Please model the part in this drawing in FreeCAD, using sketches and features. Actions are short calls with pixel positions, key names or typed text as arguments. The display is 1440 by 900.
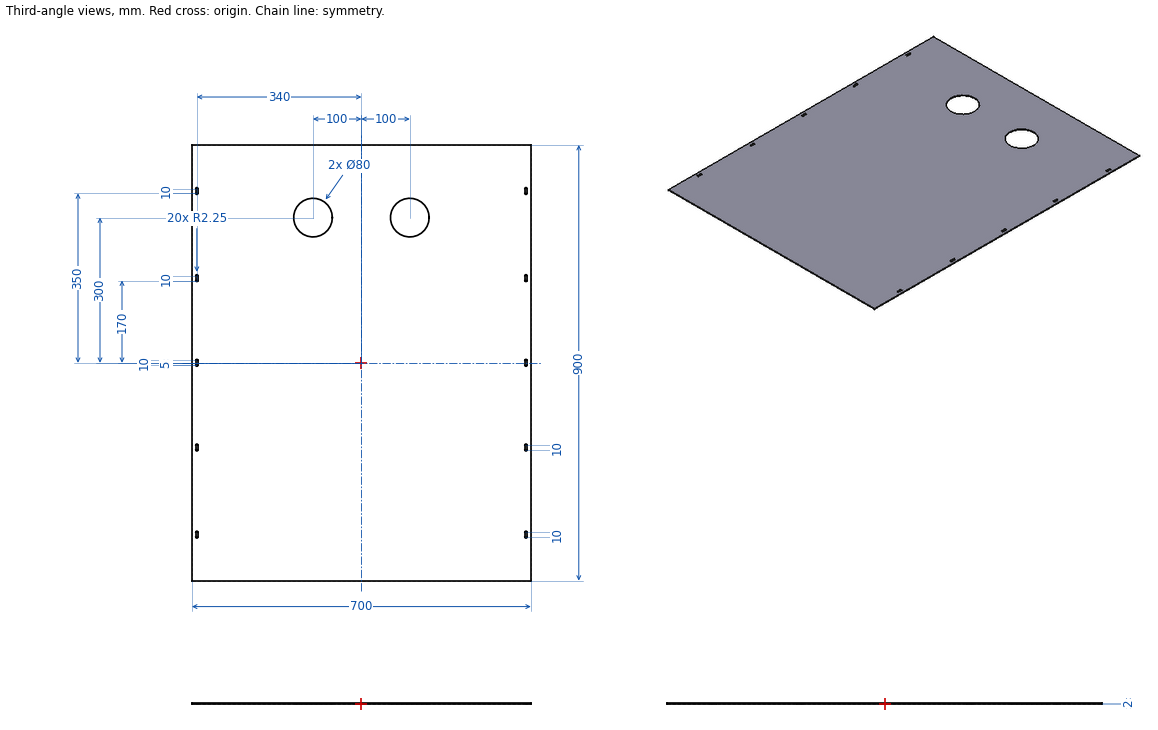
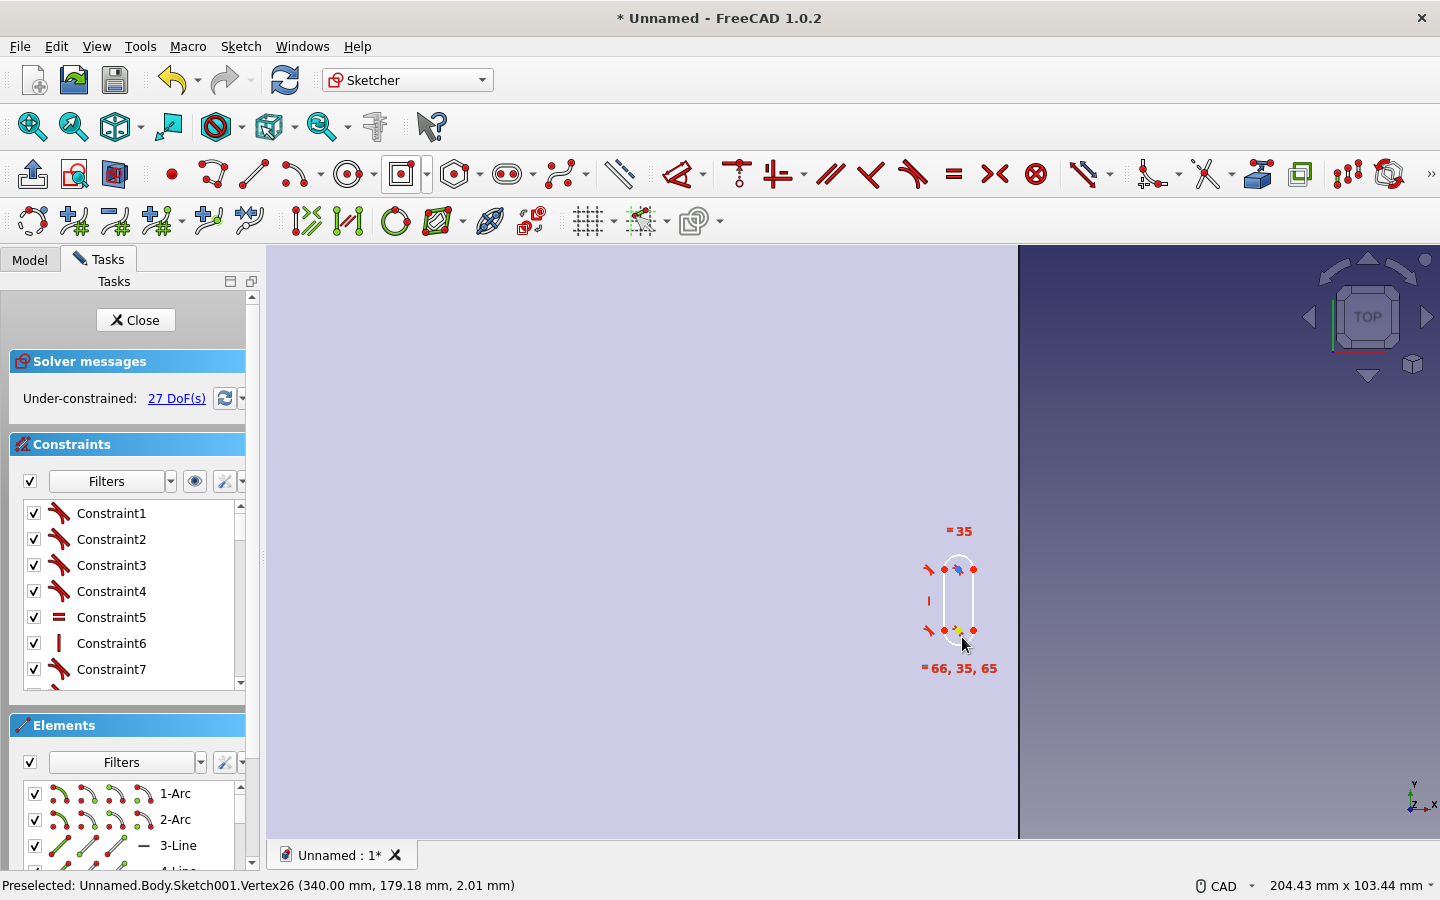
click(959, 631)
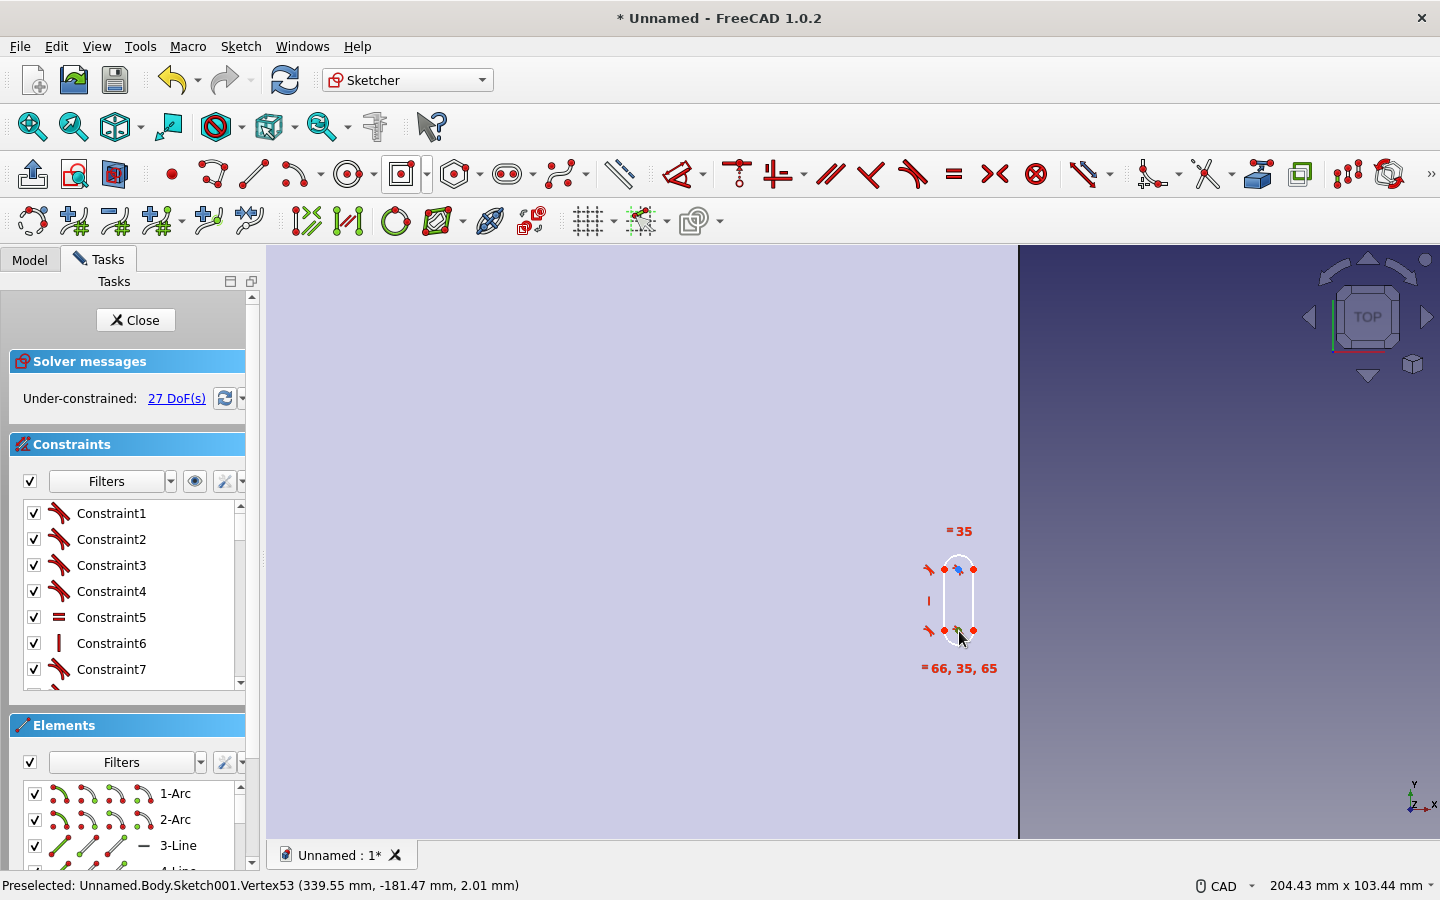
scroll(962, 637, down, 12)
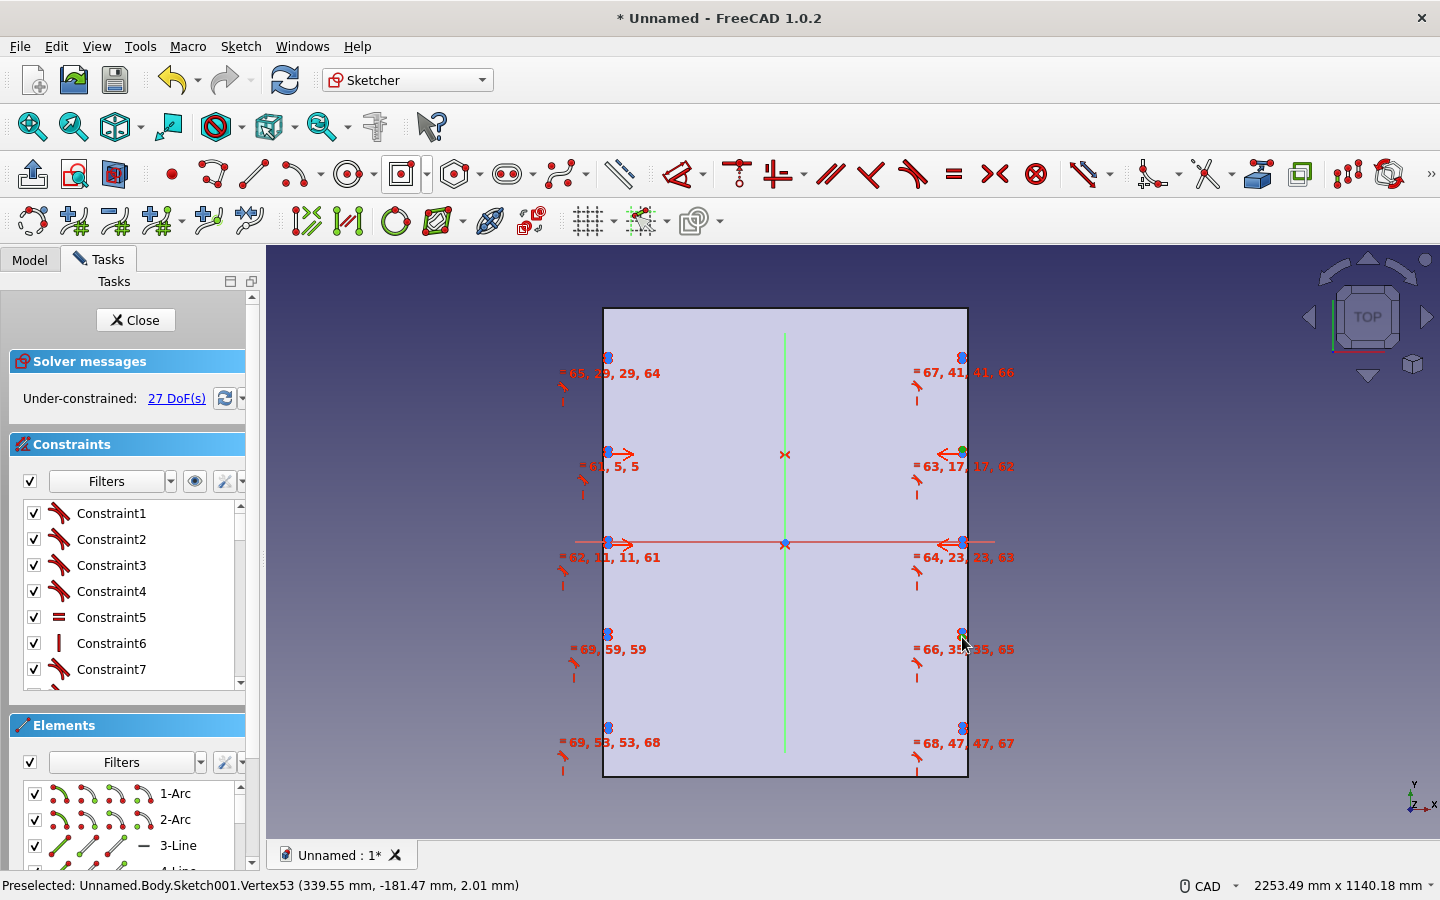
click(574, 542)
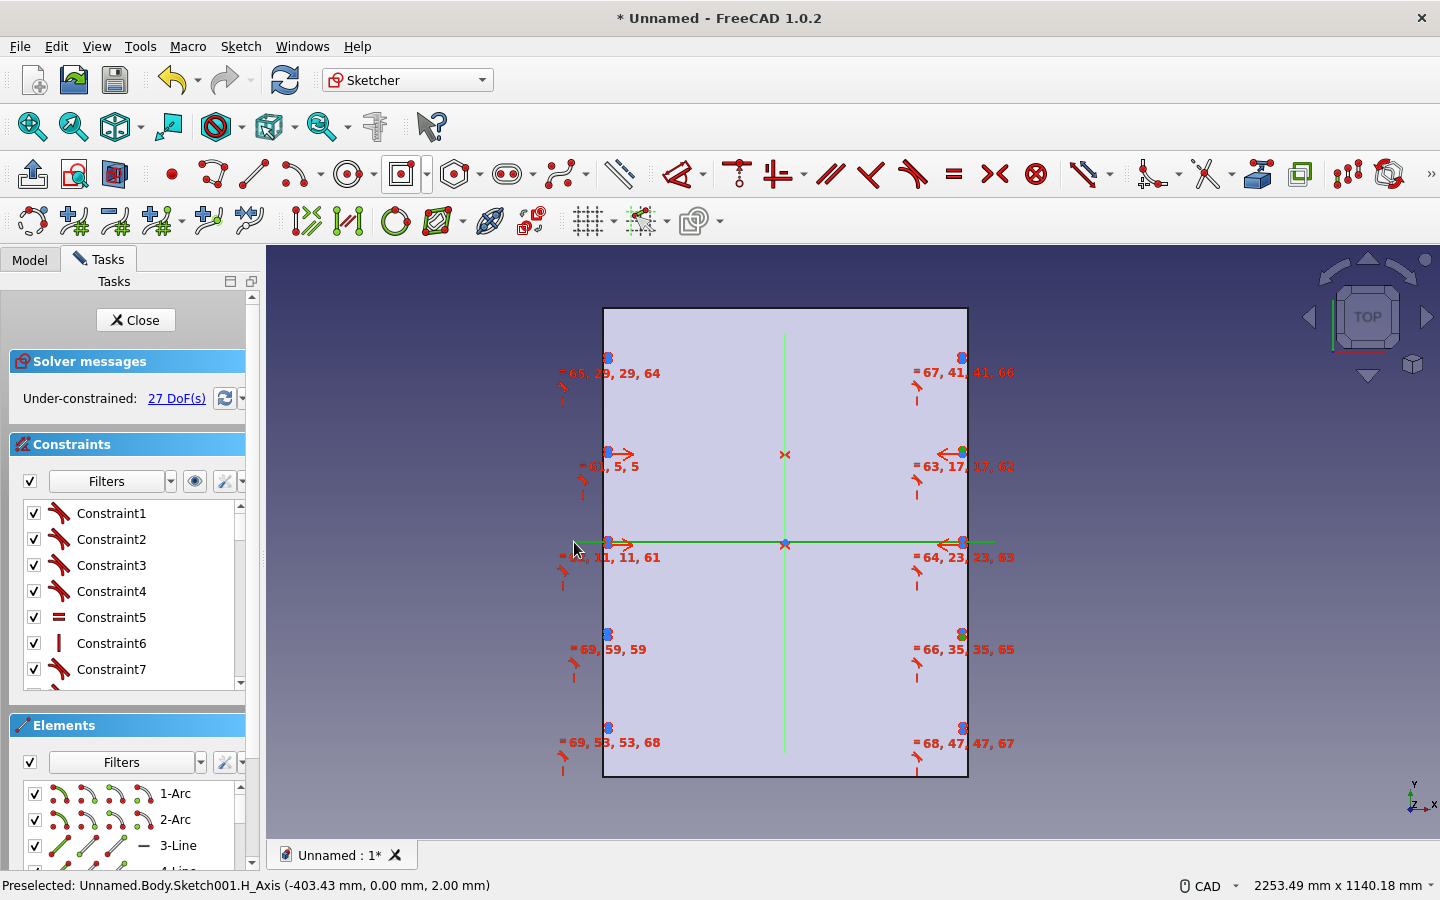
click(995, 174)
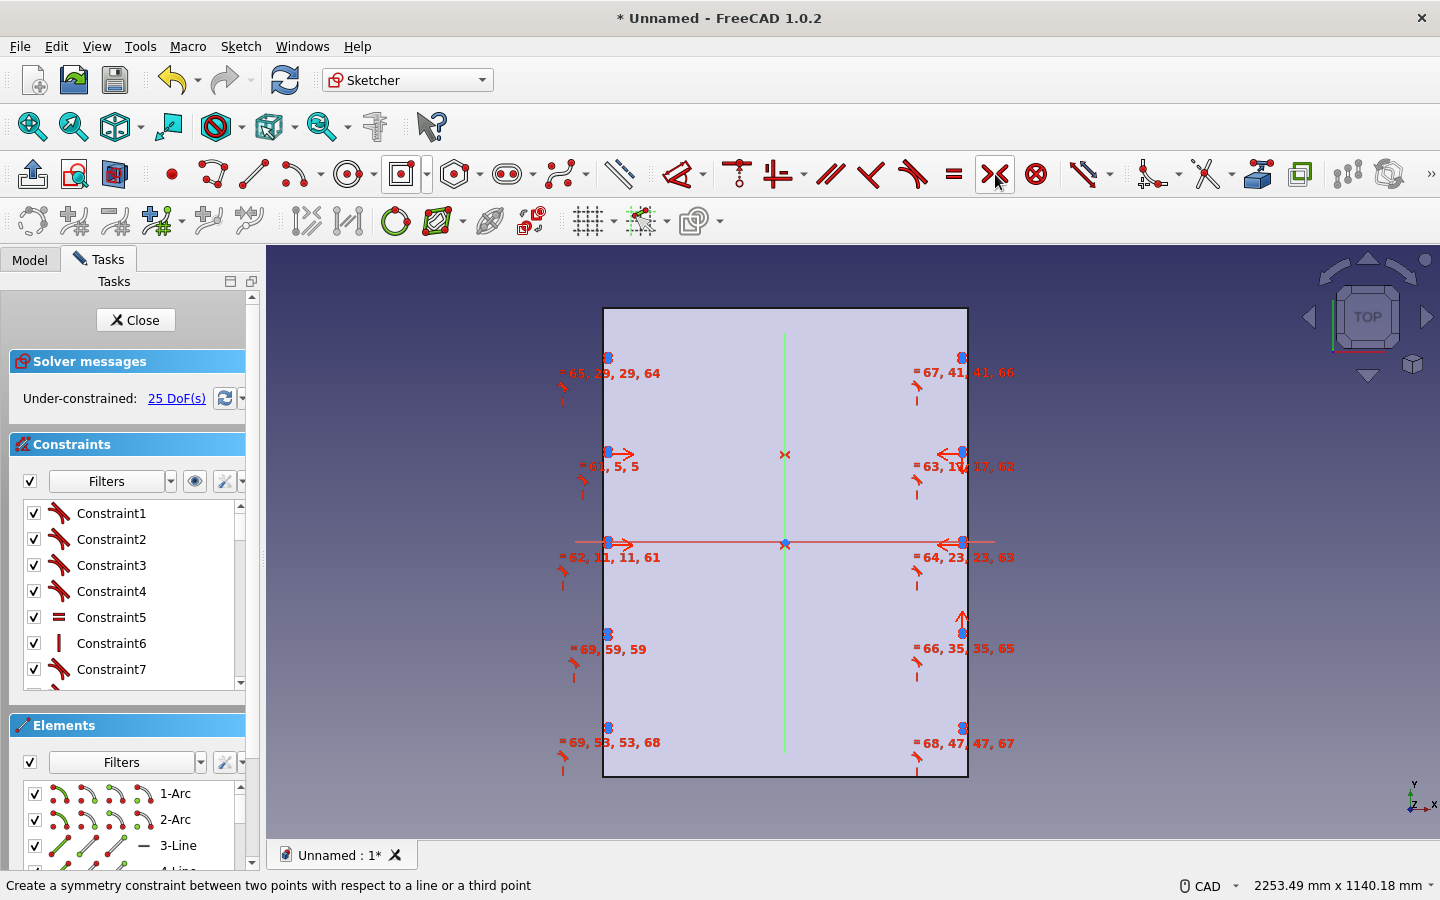
scroll(608, 361, up, 12)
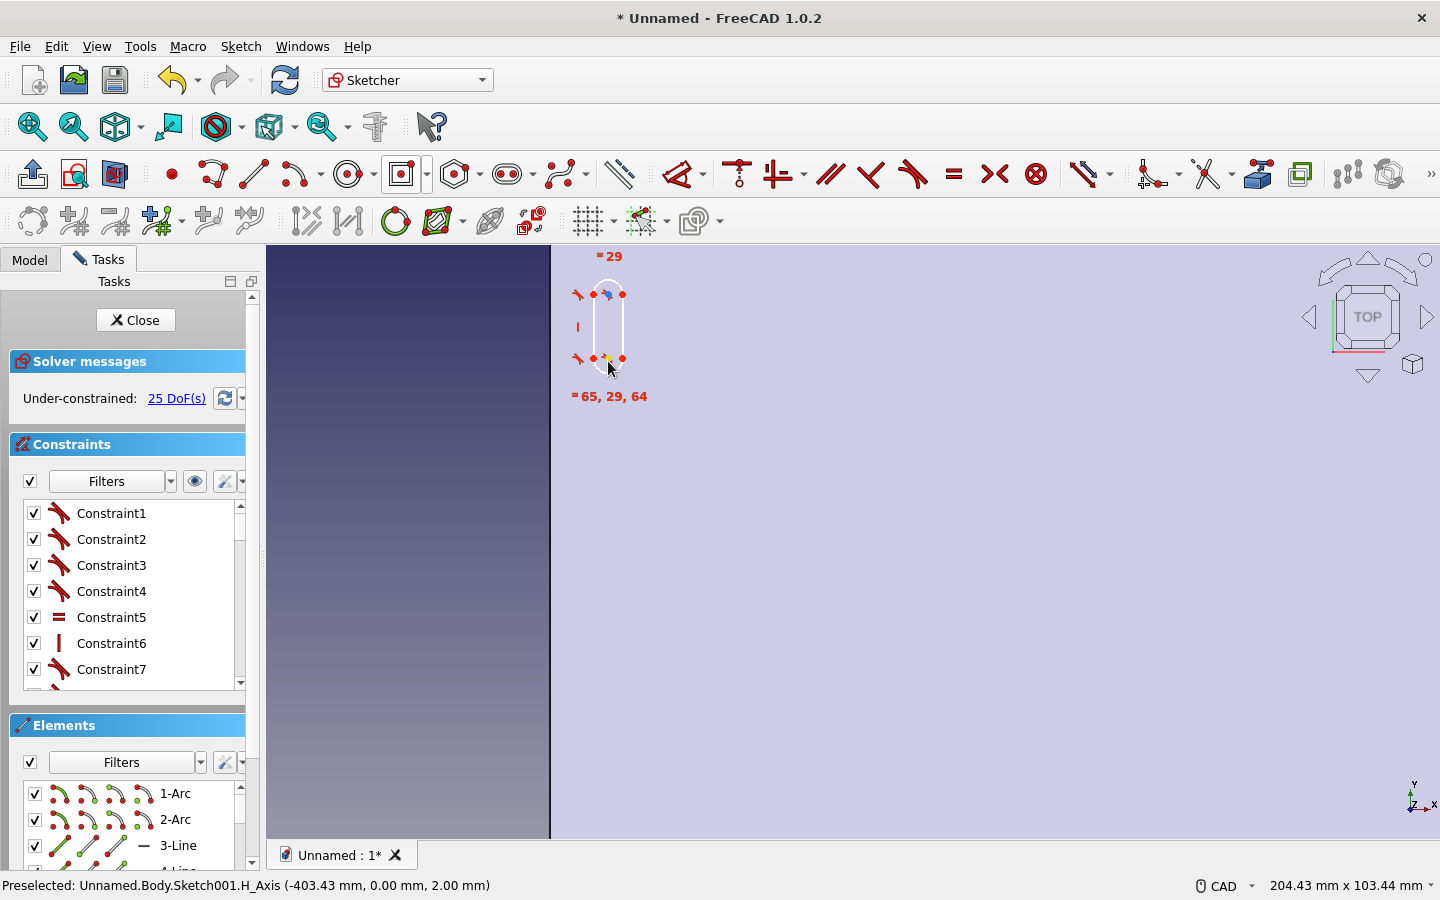
click(608, 359)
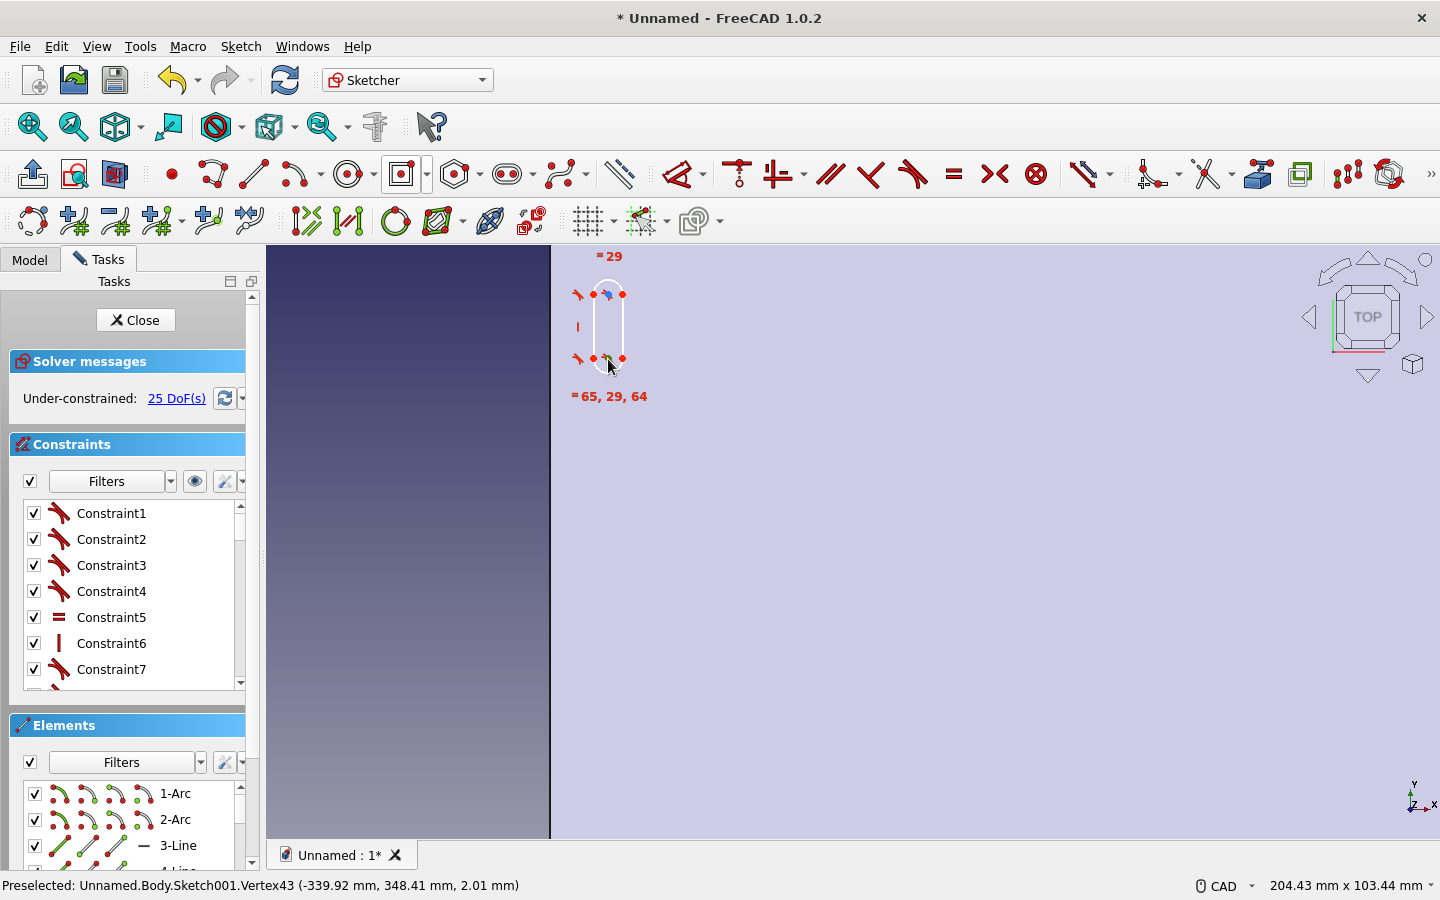
scroll(607, 361, down, 12)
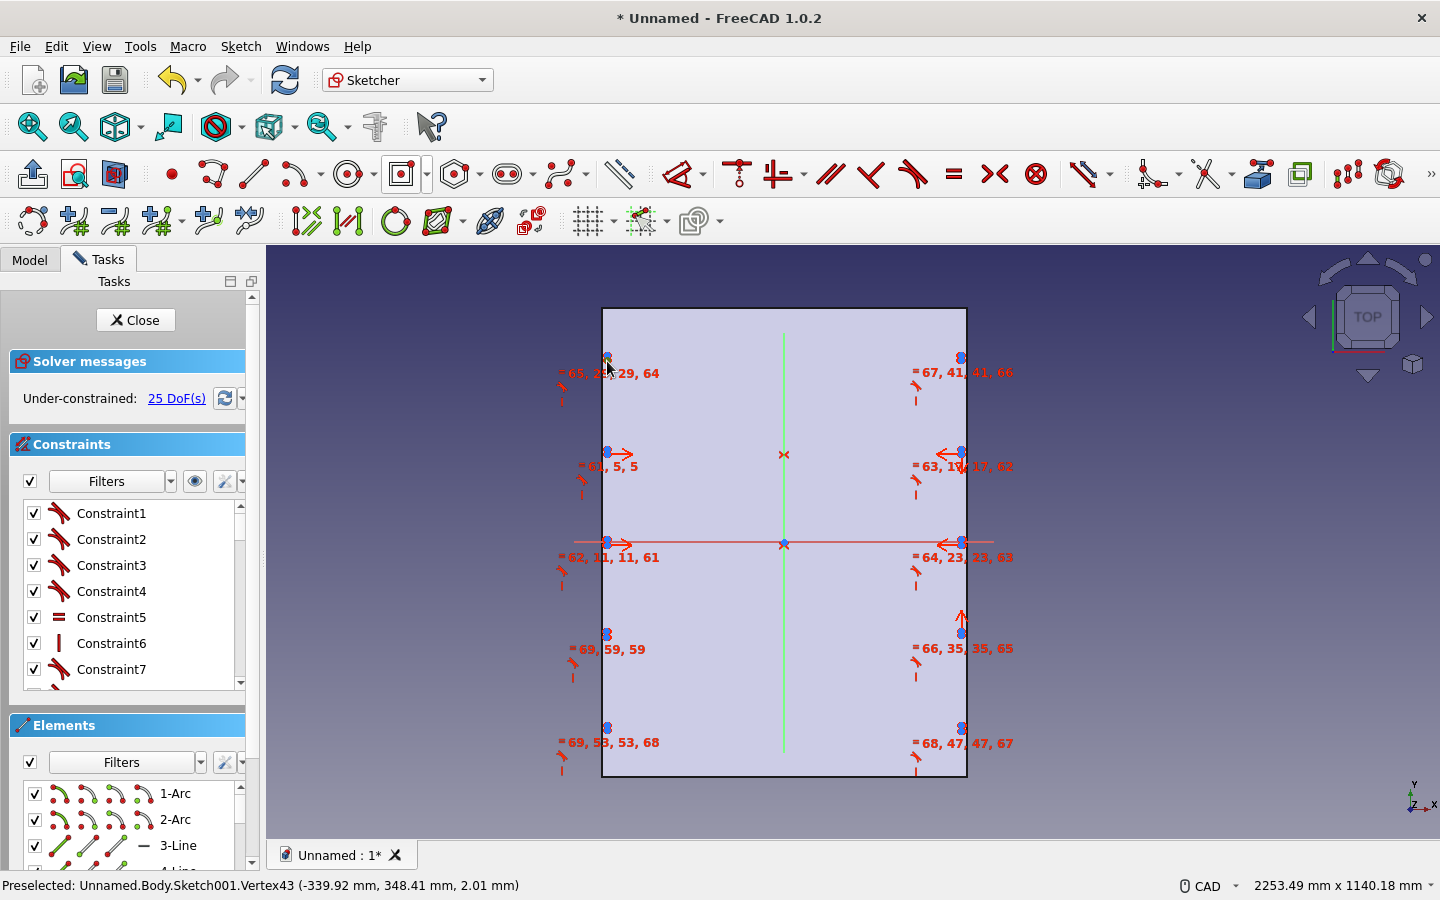
scroll(961, 361, up, 12)